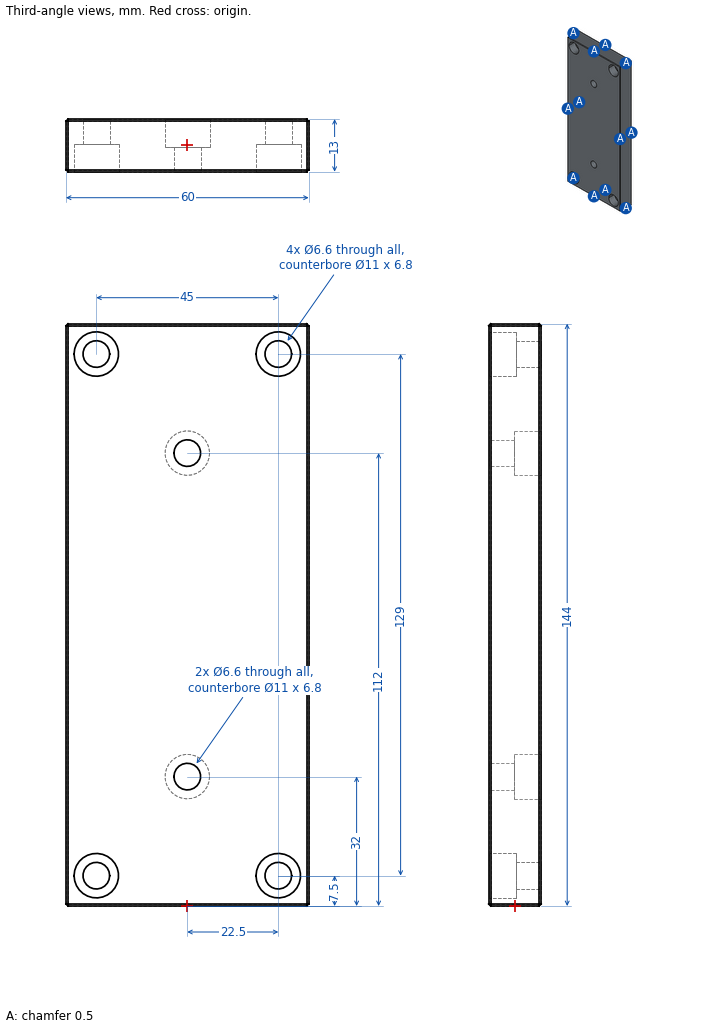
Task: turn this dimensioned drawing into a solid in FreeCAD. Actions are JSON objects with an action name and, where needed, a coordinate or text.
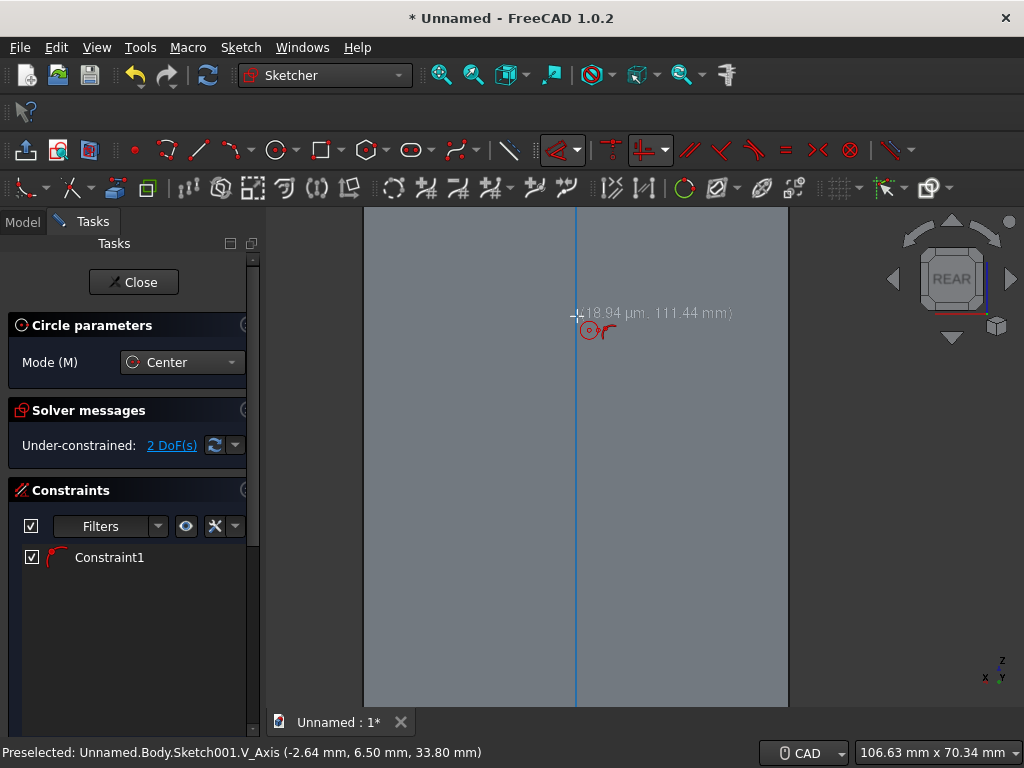
{"action": "left_click", "coordinate": [576, 314]}
{"action": "left_click", "coordinate": [593, 298]}
{"action": "key", "text": "Escape"}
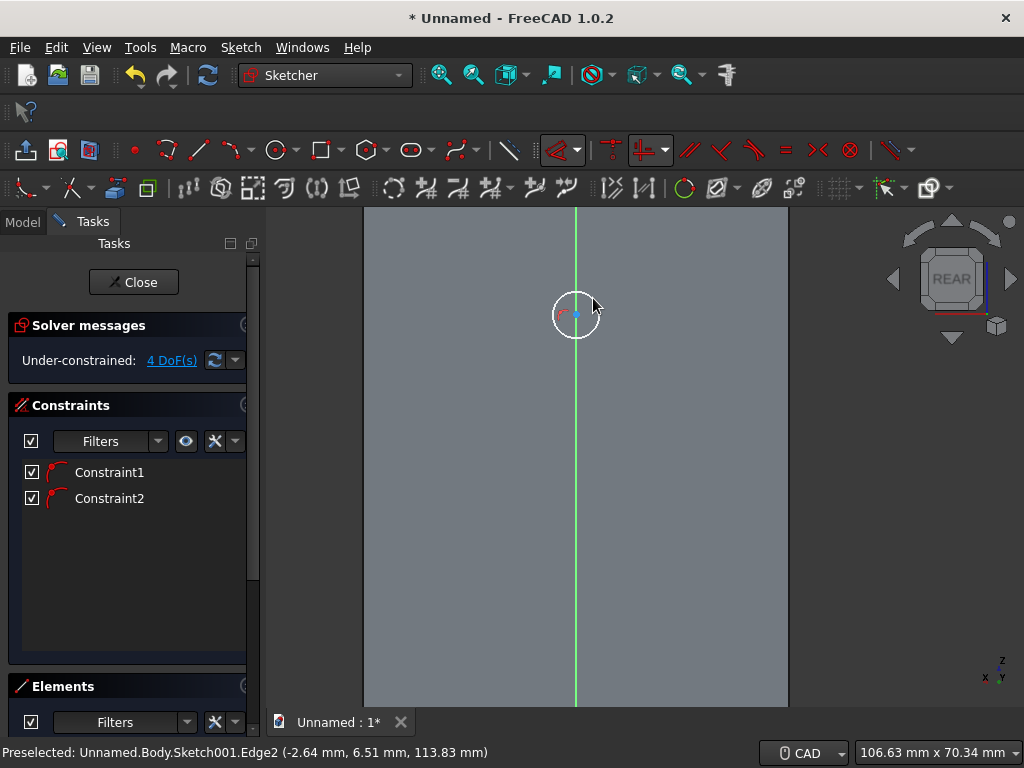
{"action": "scroll", "coordinate": [577, 315], "scroll_direction": "down", "scroll_amount": 5}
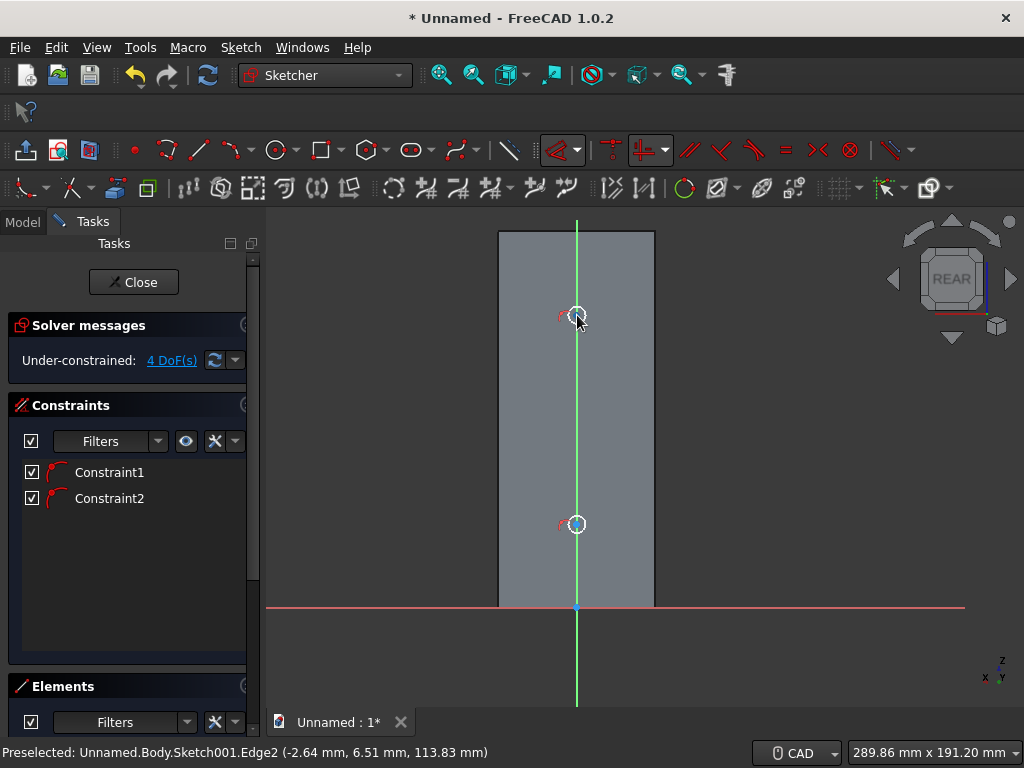
{"action": "scroll", "coordinate": [583, 518], "scroll_direction": "up", "scroll_amount": 5}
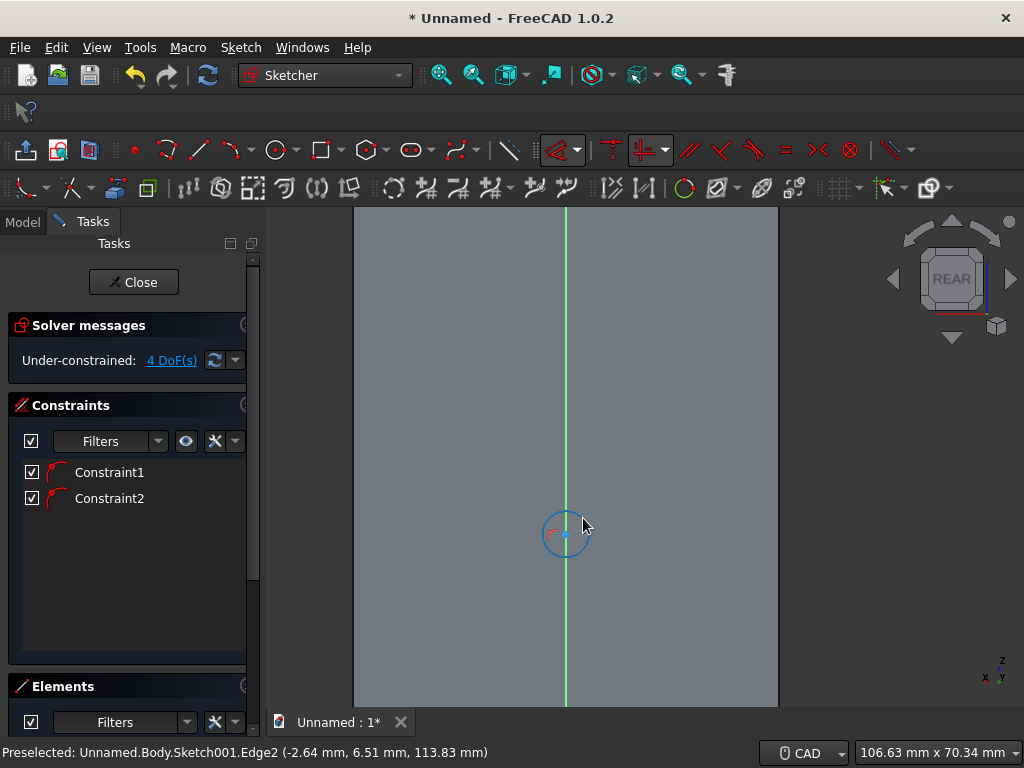
{"action": "left_click", "coordinate": [582, 518]}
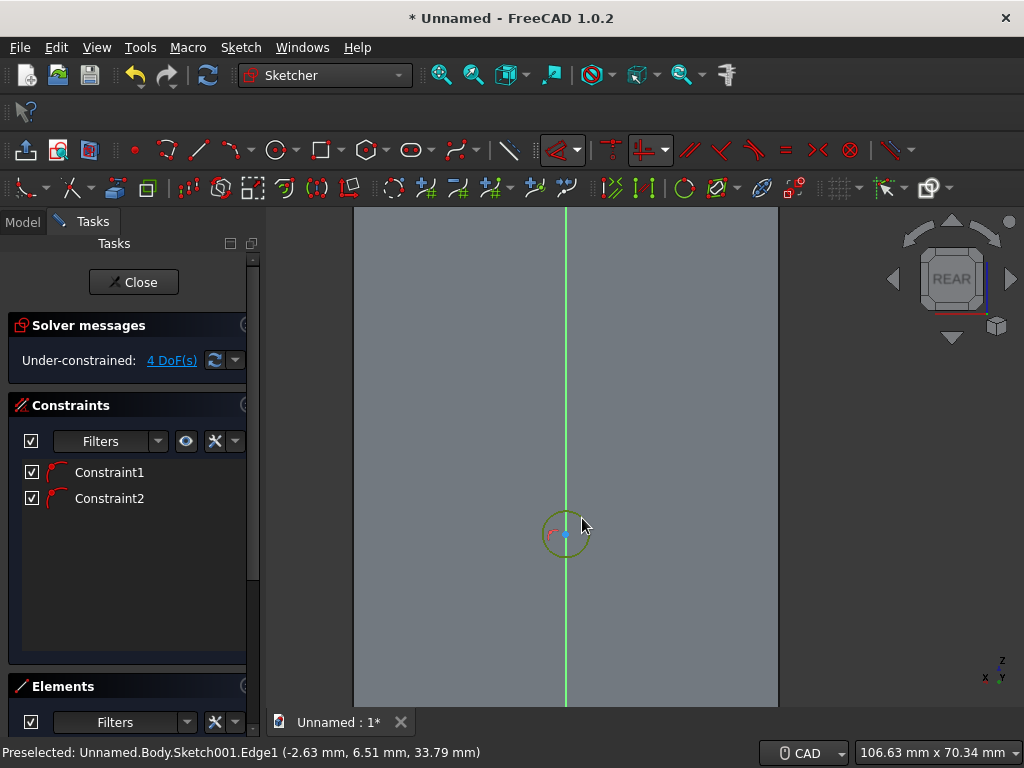
{"action": "scroll", "coordinate": [583, 519], "scroll_direction": "down", "scroll_amount": 5}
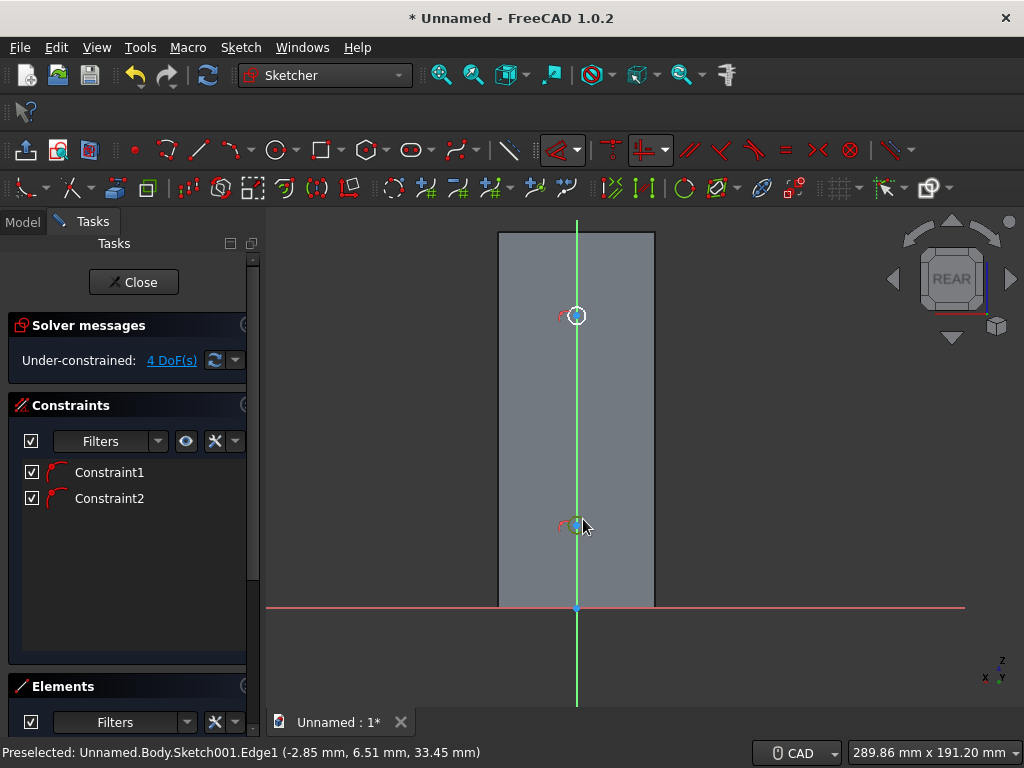
{"action": "scroll", "coordinate": [583, 310], "scroll_direction": "up", "scroll_amount": 5}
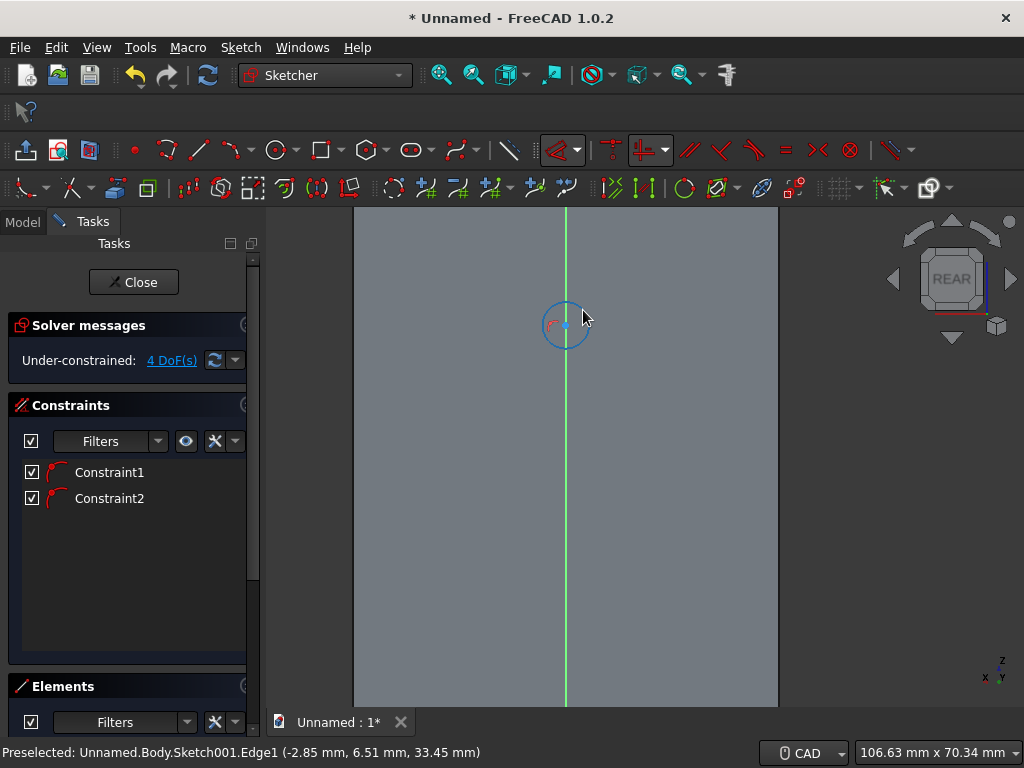
{"action": "left_click", "coordinate": [582, 309]}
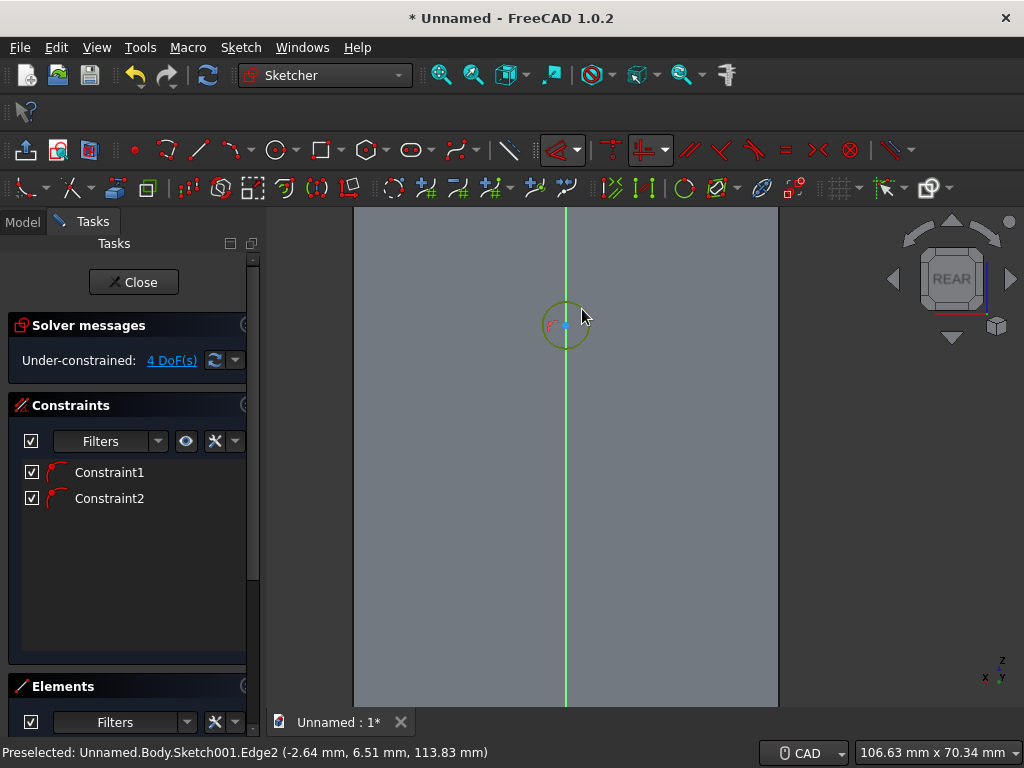
{"action": "key", "text": "e"}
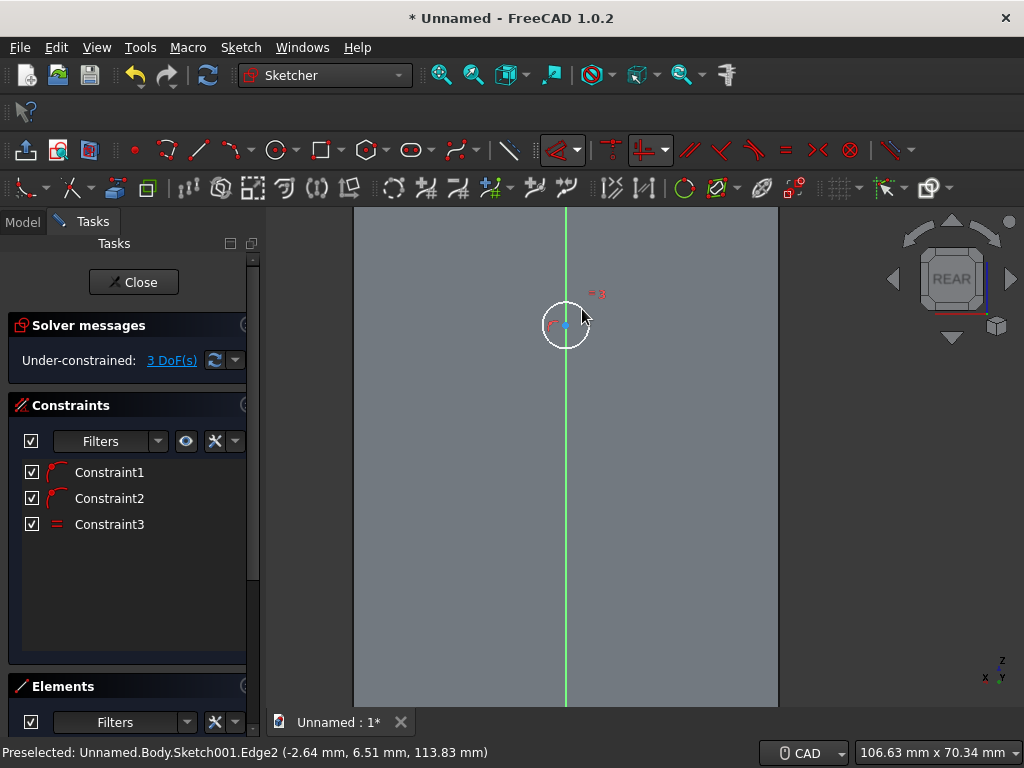
{"action": "scroll", "coordinate": [583, 309], "scroll_direction": "down", "scroll_amount": 5}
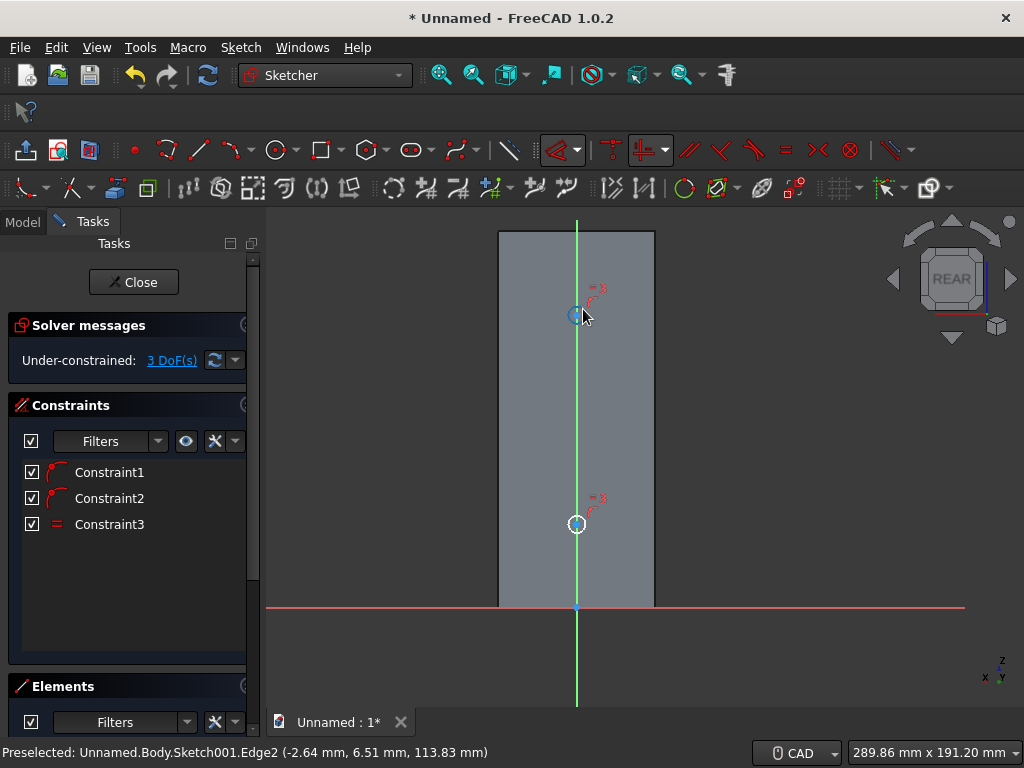
{"action": "scroll", "coordinate": [583, 518], "scroll_direction": "up", "scroll_amount": 5}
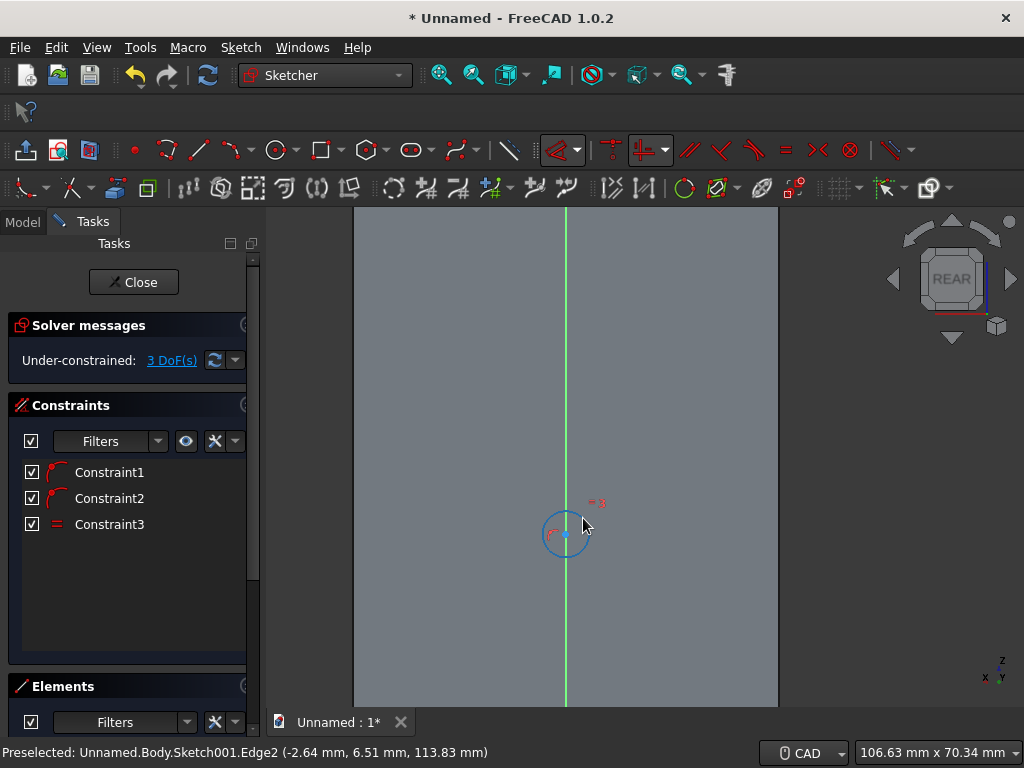
{"action": "left_click", "coordinate": [582, 518]}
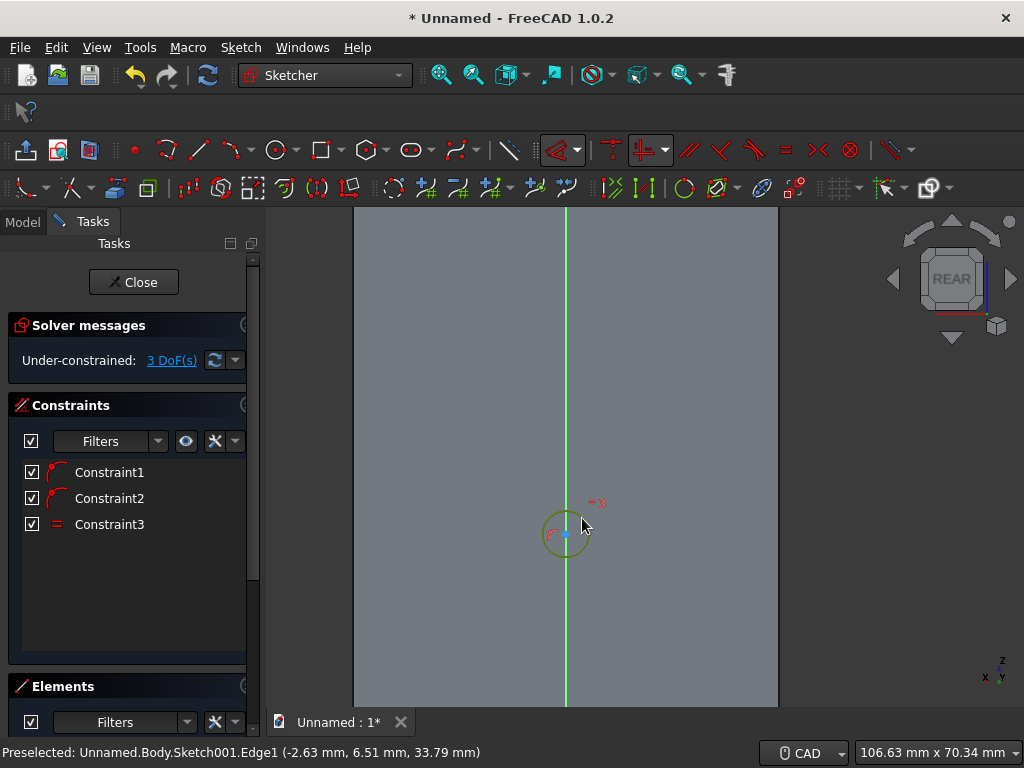
{"action": "key", "text": "k o"}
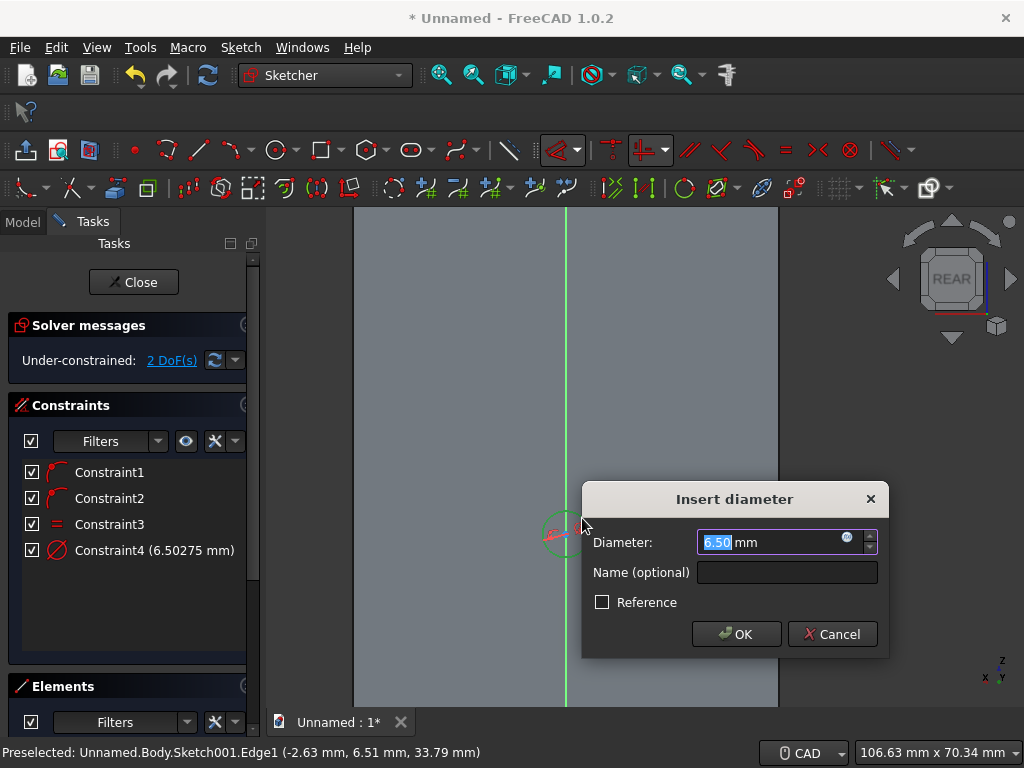
{"action": "type", "text": "6.6"}
{"action": "key", "text": "Return"}